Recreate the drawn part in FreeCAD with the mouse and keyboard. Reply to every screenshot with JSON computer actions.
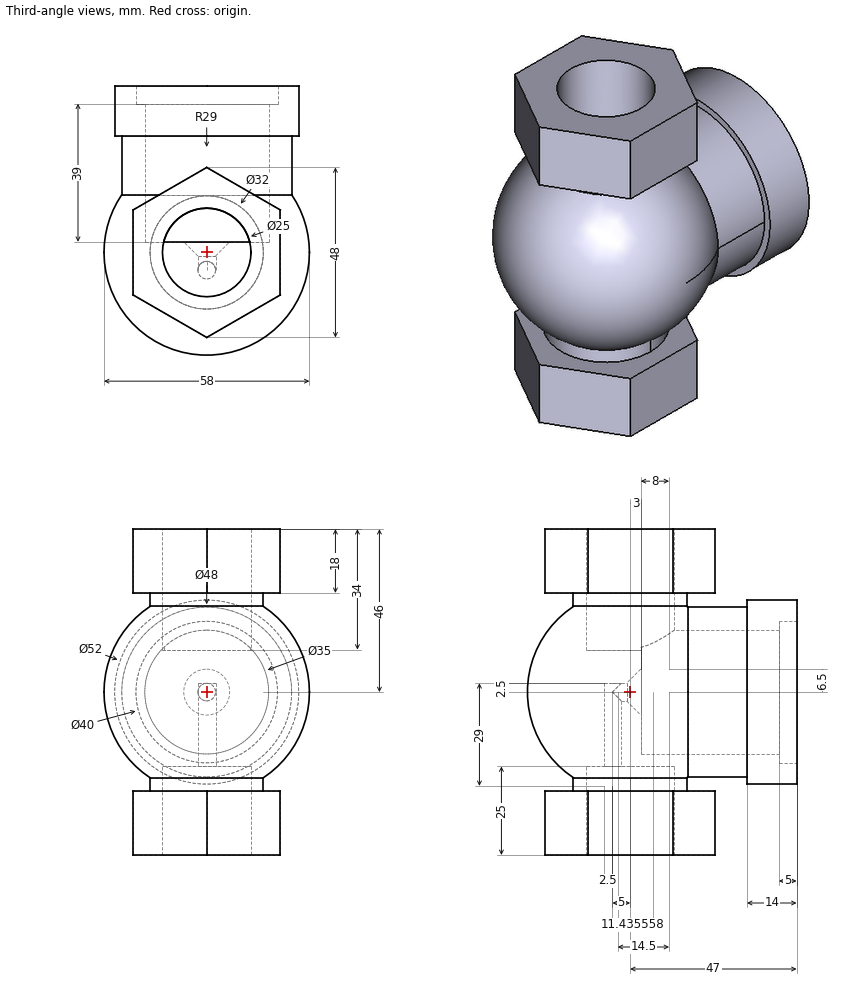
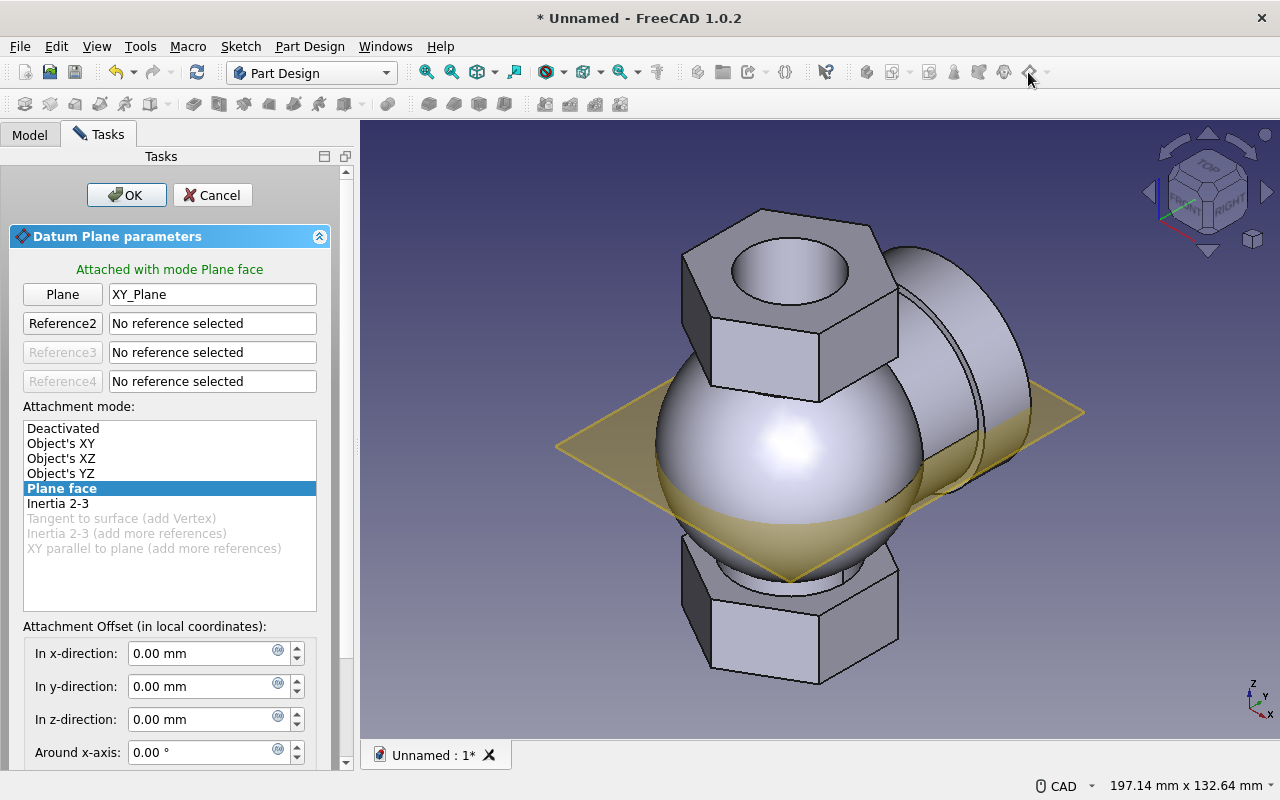
{"action": "triple_click", "coordinate": [210, 720]}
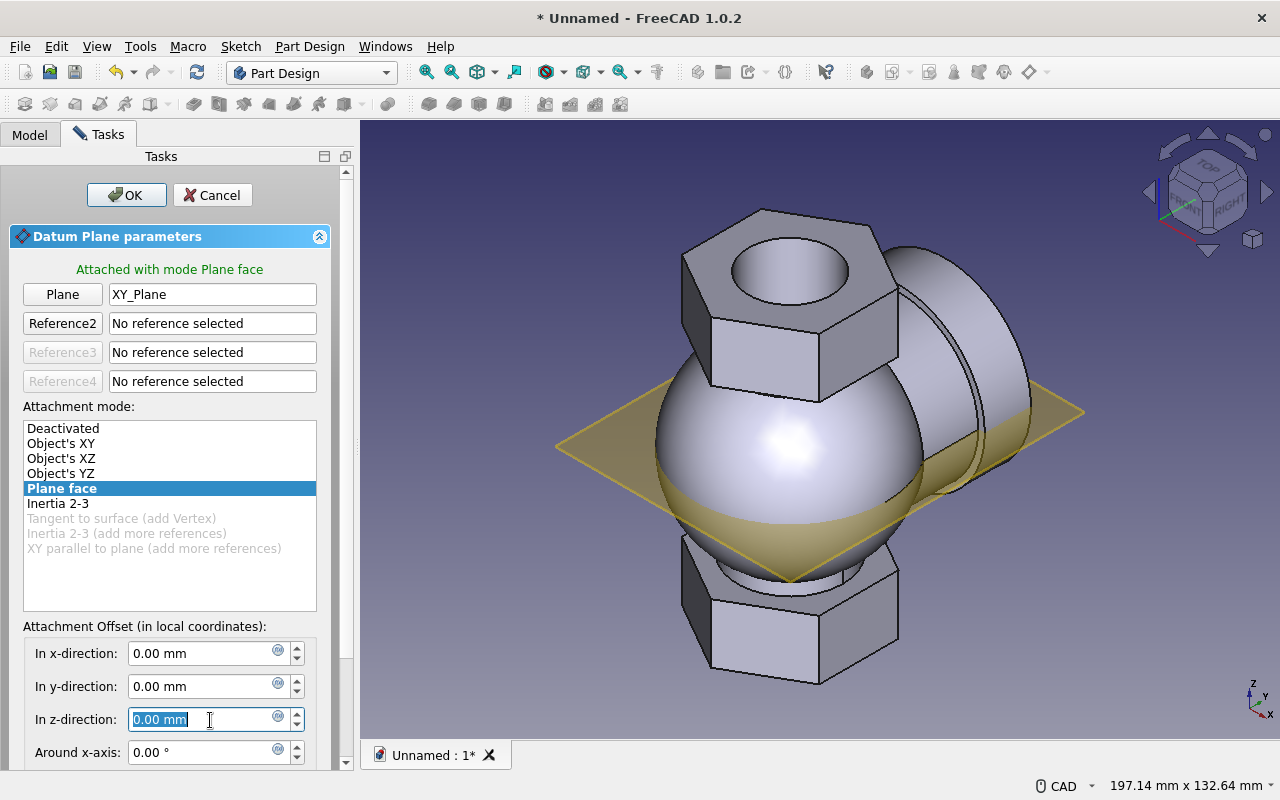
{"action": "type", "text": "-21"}
{"action": "key", "text": "Tab"}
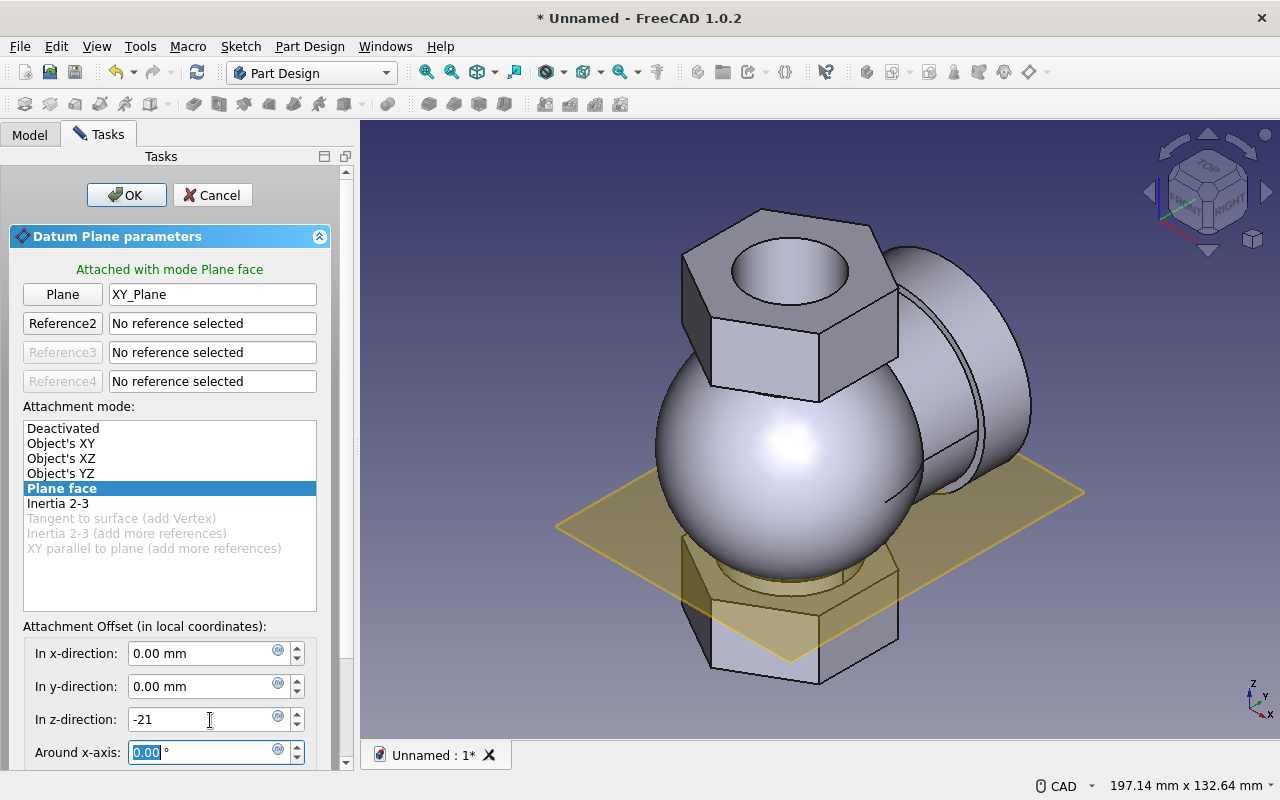
{"action": "left_click", "coordinate": [127, 195]}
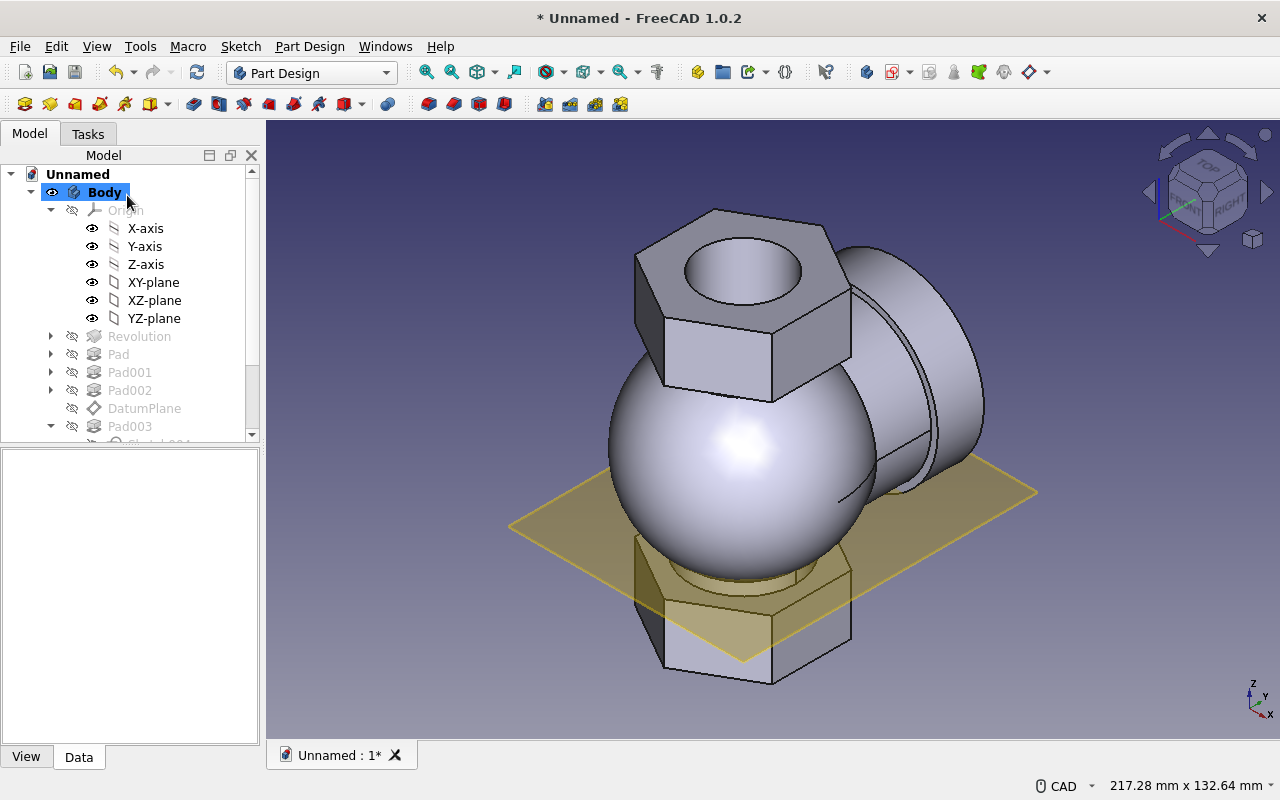
{"action": "scroll", "coordinate": [101, 296], "scroll_direction": "down", "scroll_amount": 3}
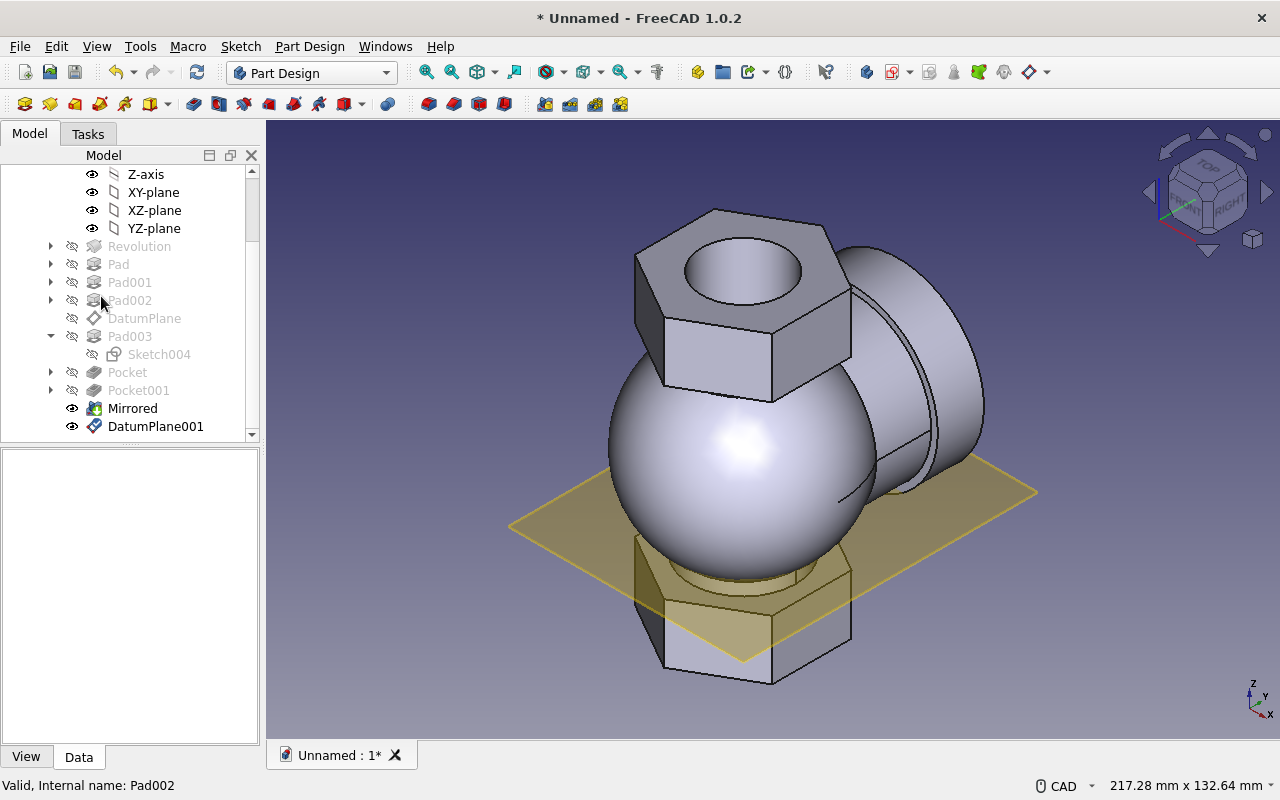
{"action": "left_click", "coordinate": [117, 426]}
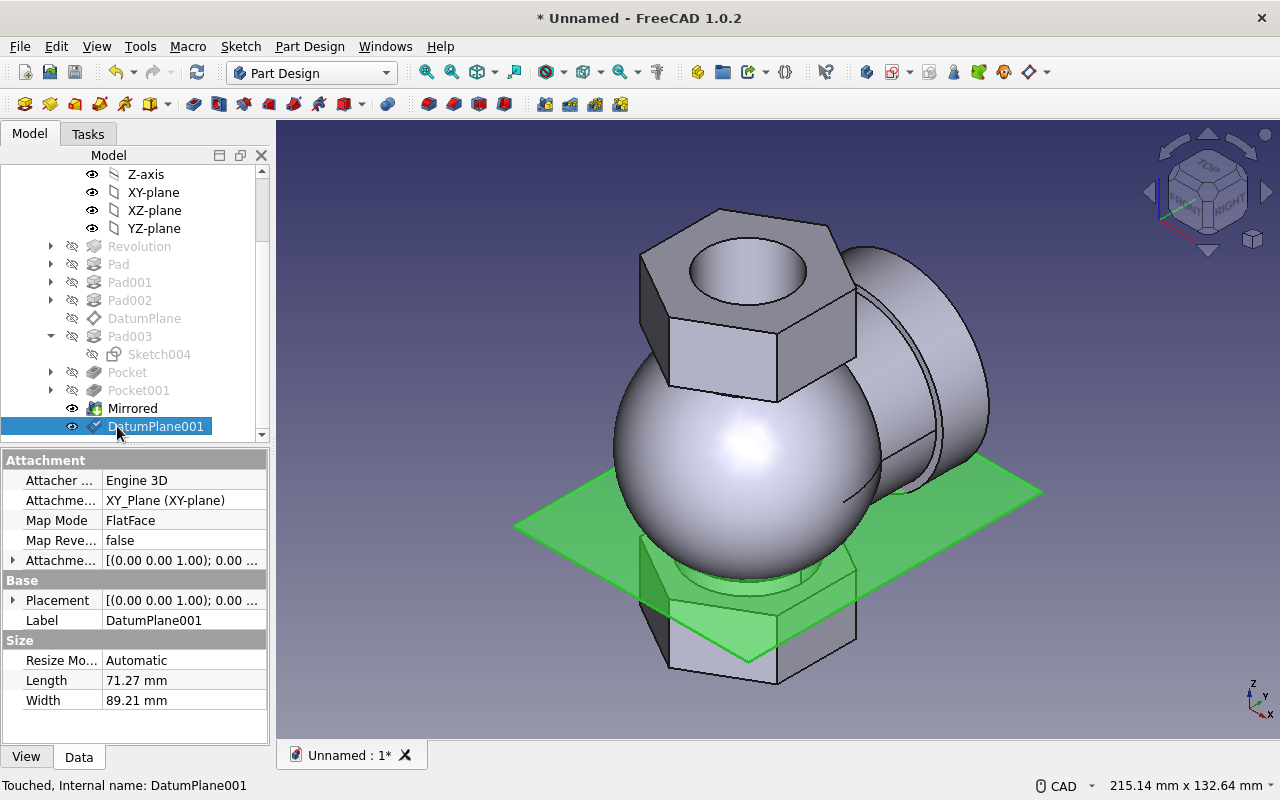
{"action": "left_click", "coordinate": [892, 72]}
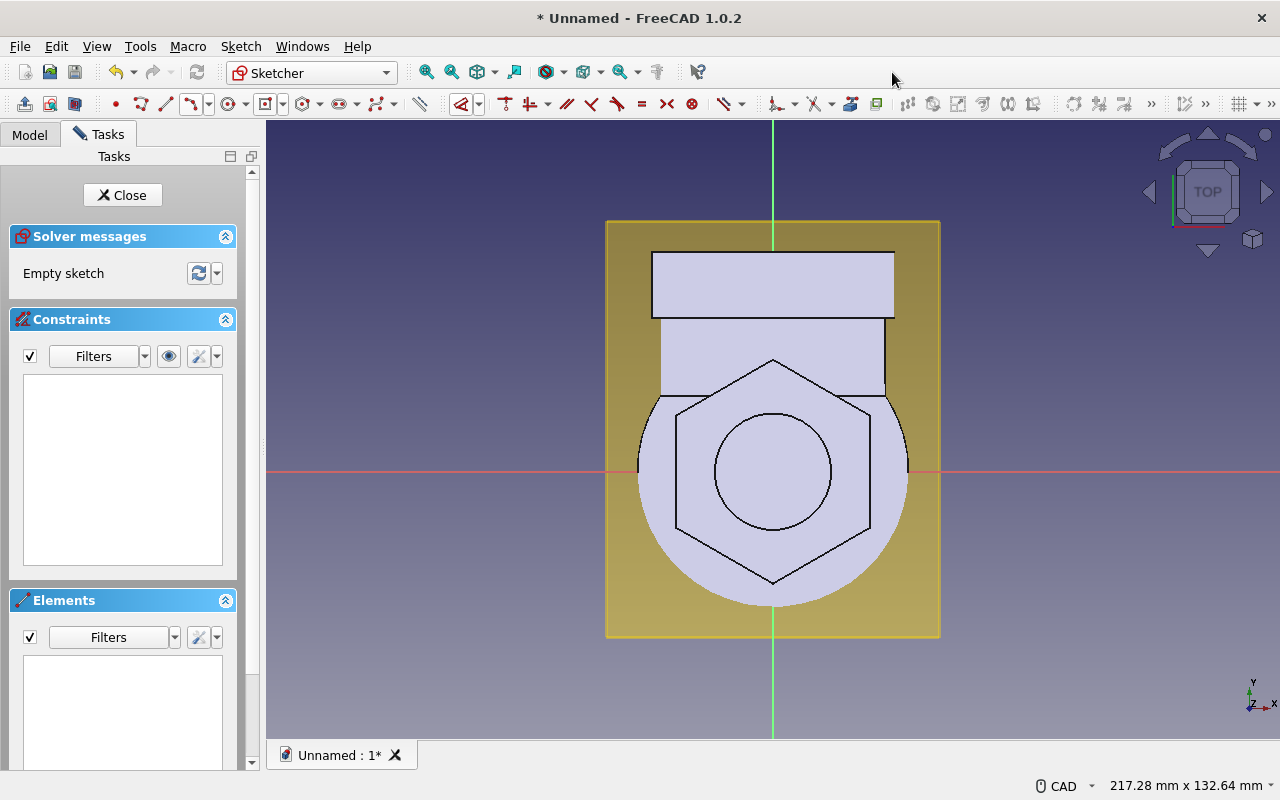
{"action": "left_click", "coordinate": [75, 104]}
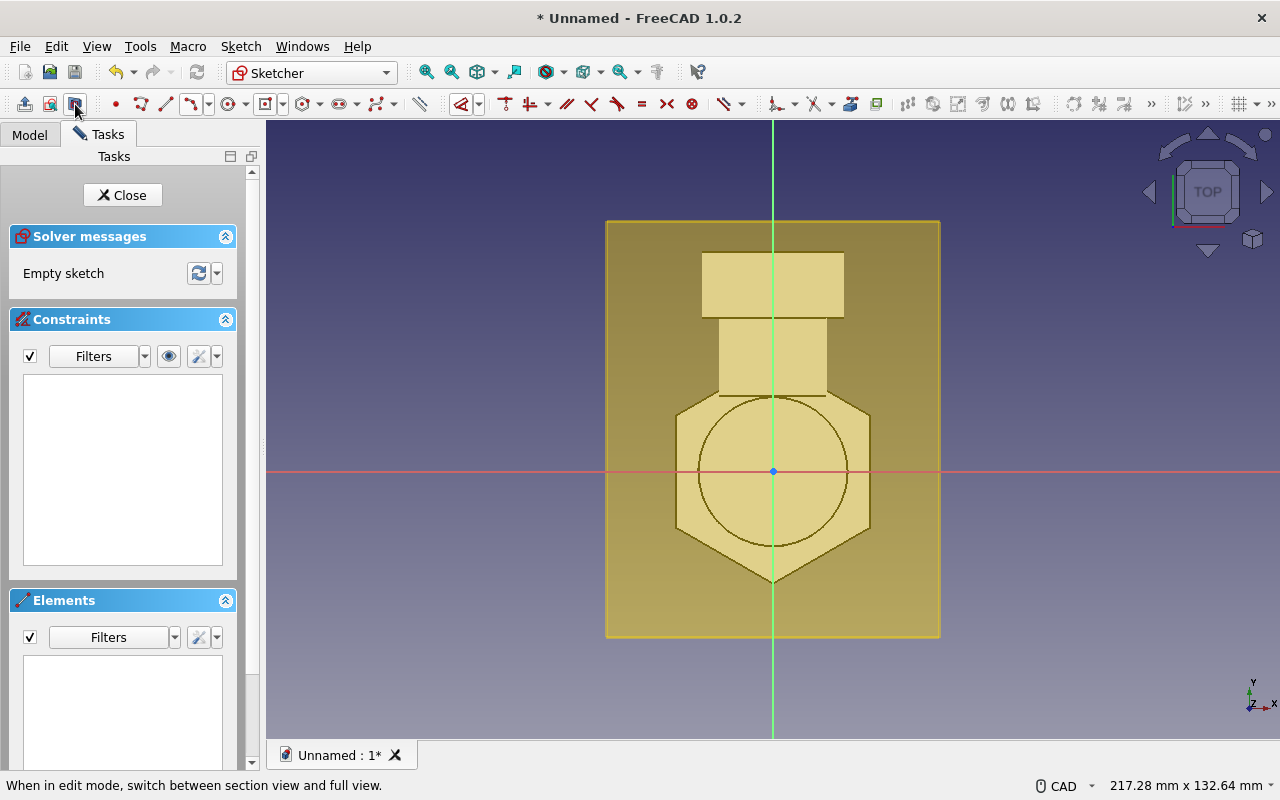
{"action": "scroll", "coordinate": [803, 490], "scroll_direction": "up", "scroll_amount": 6}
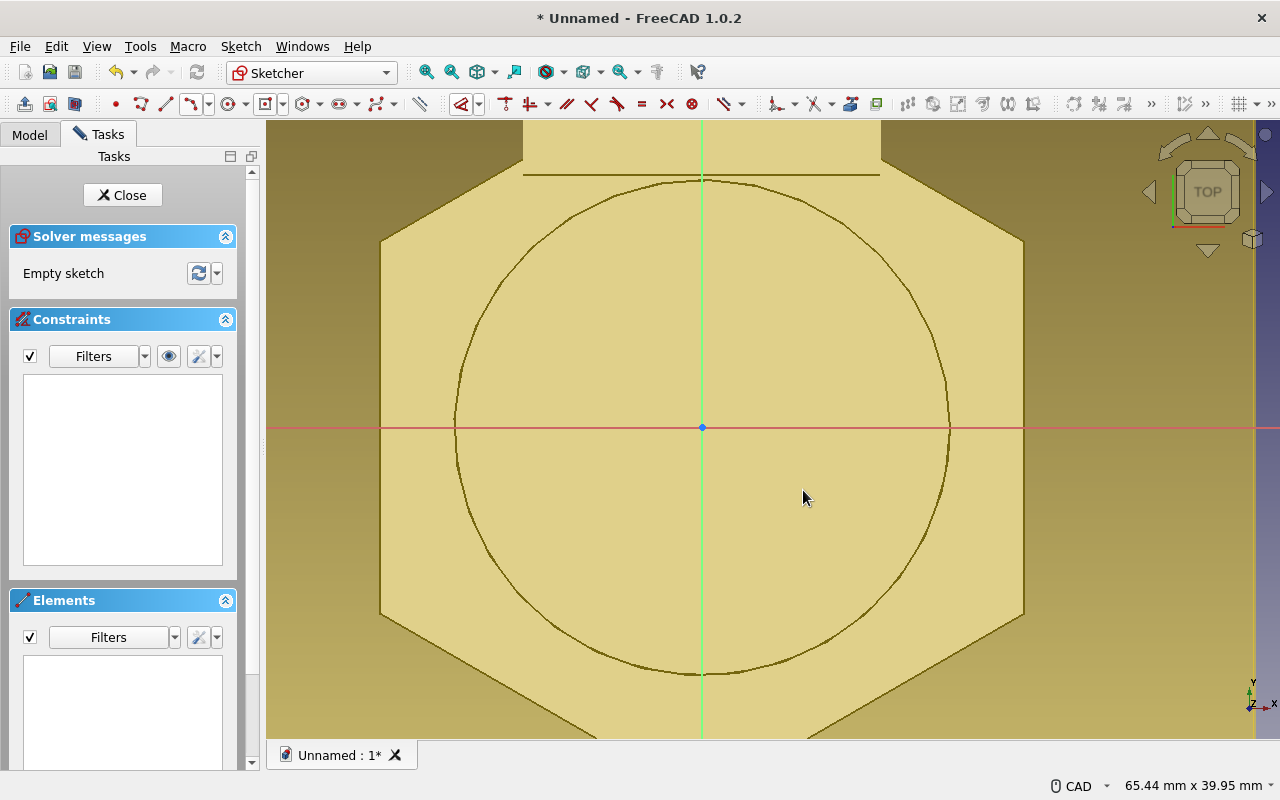
{"action": "key", "text": "g c"}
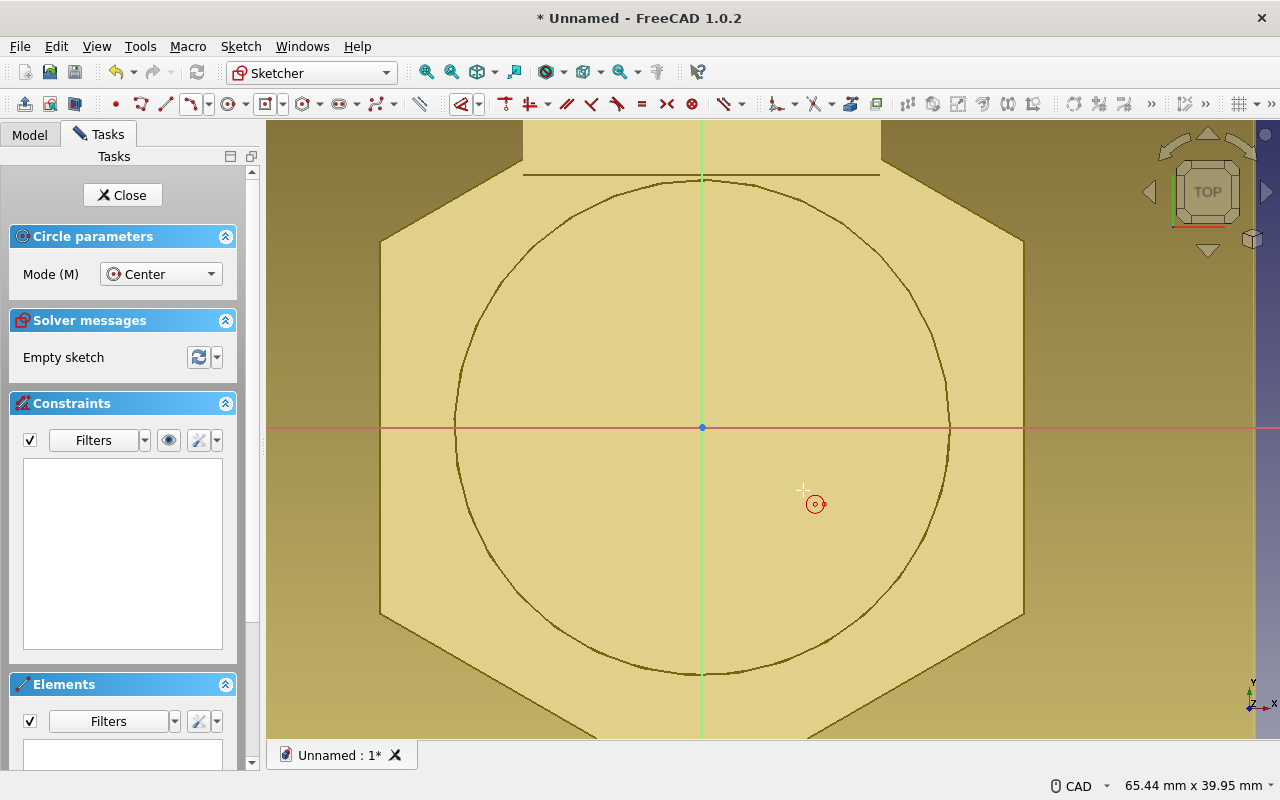
{"action": "left_click", "coordinate": [702, 428]}
{"action": "left_click", "coordinate": [839, 291]}
{"action": "key", "text": "Escape"}